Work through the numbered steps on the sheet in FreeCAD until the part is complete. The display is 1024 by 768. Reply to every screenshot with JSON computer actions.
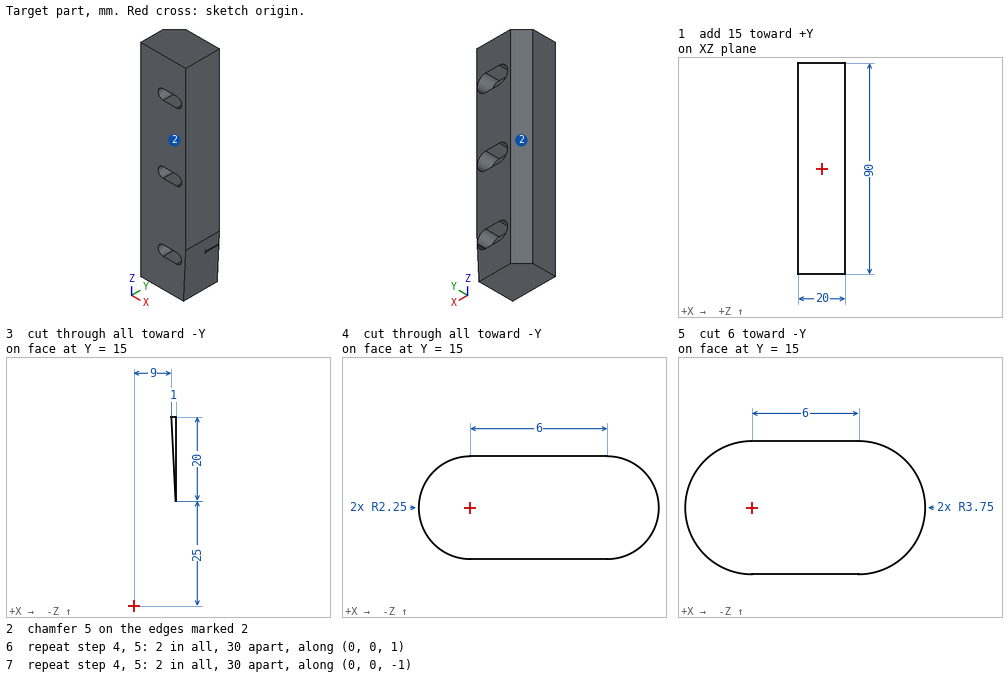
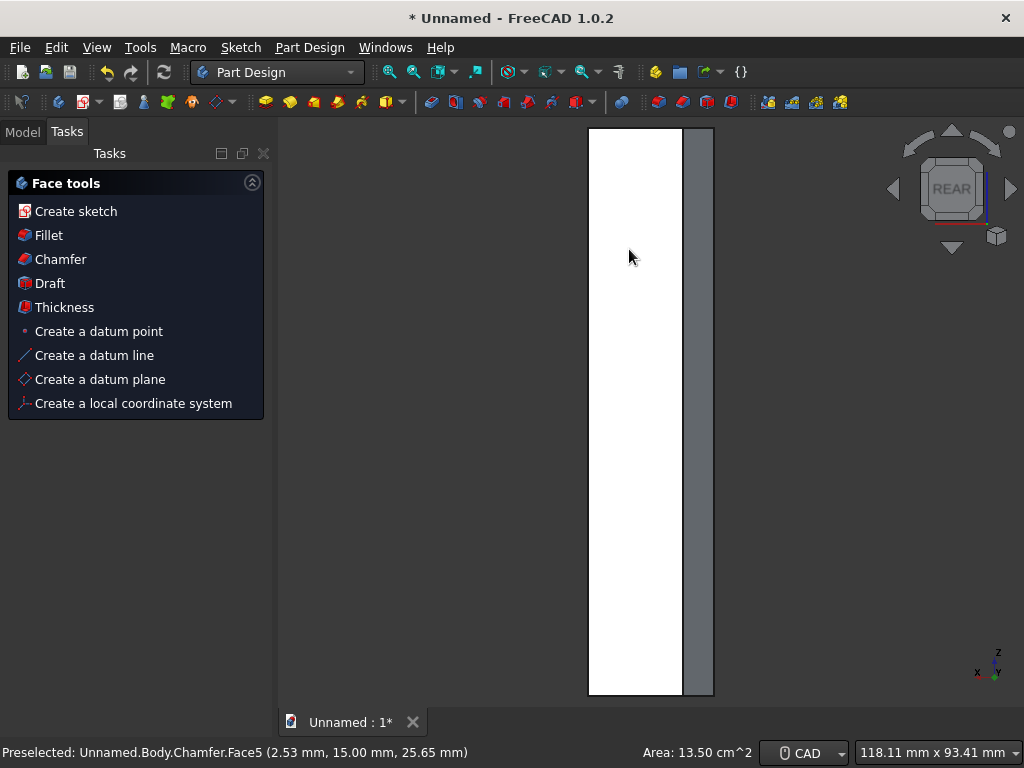
{"action": "left_click", "coordinate": [84, 102]}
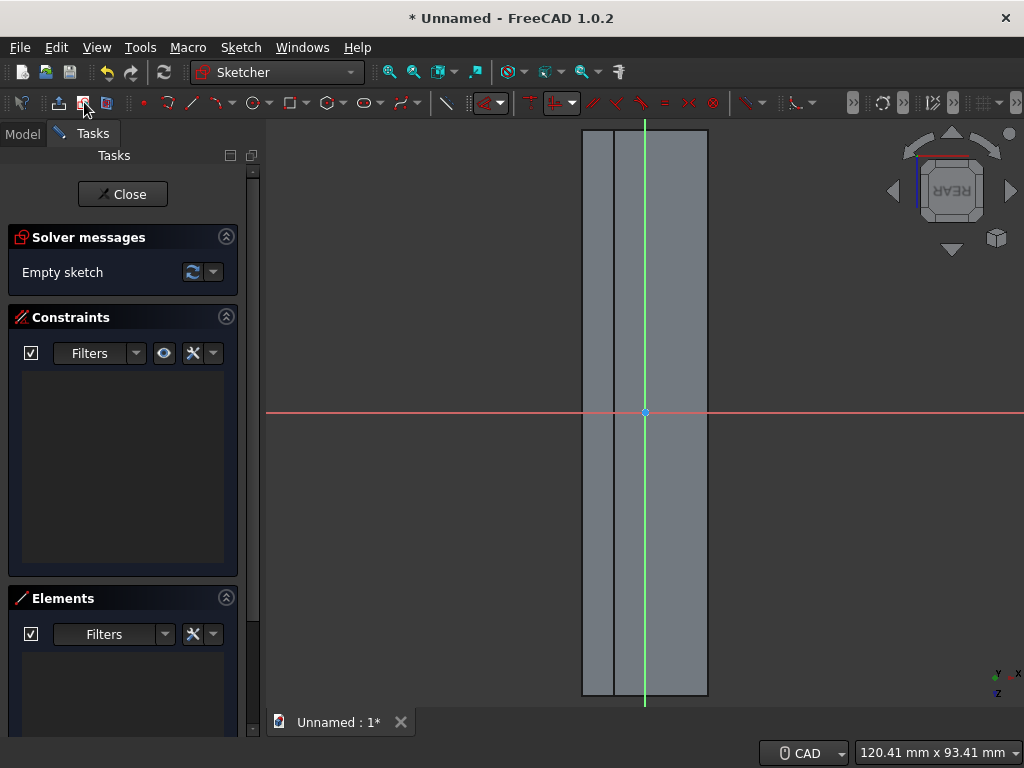
{"action": "scroll", "coordinate": [294, 679], "scroll_direction": "down", "scroll_amount": 1}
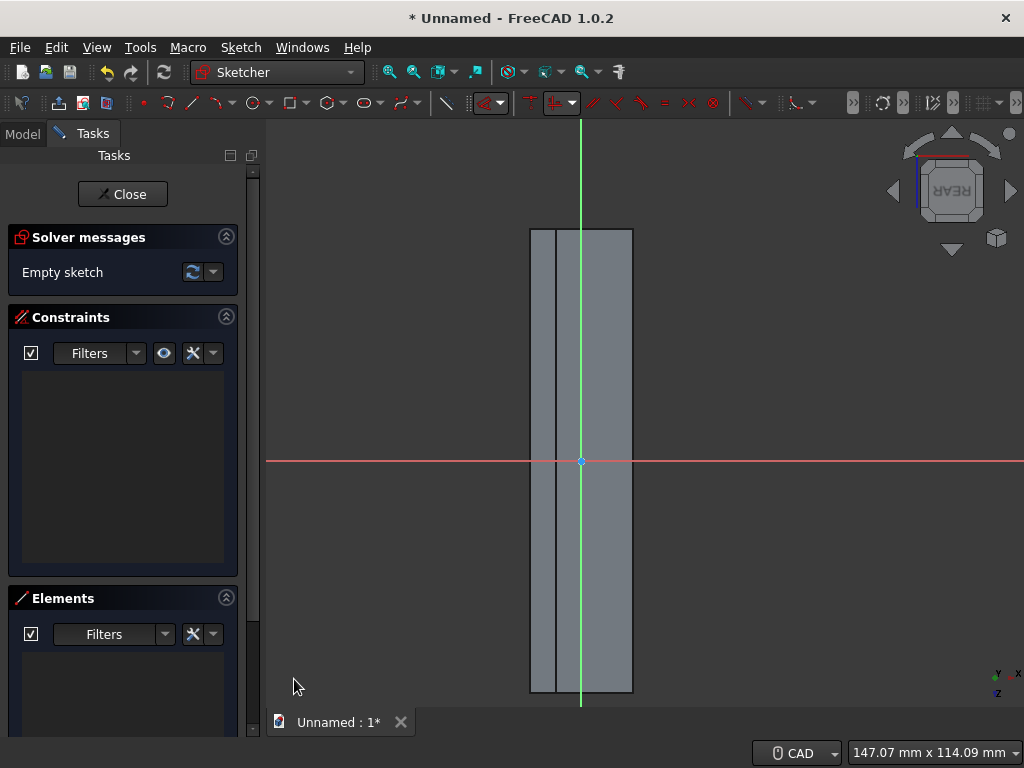
{"action": "scroll", "coordinate": [669, 208], "scroll_direction": "up", "scroll_amount": 2}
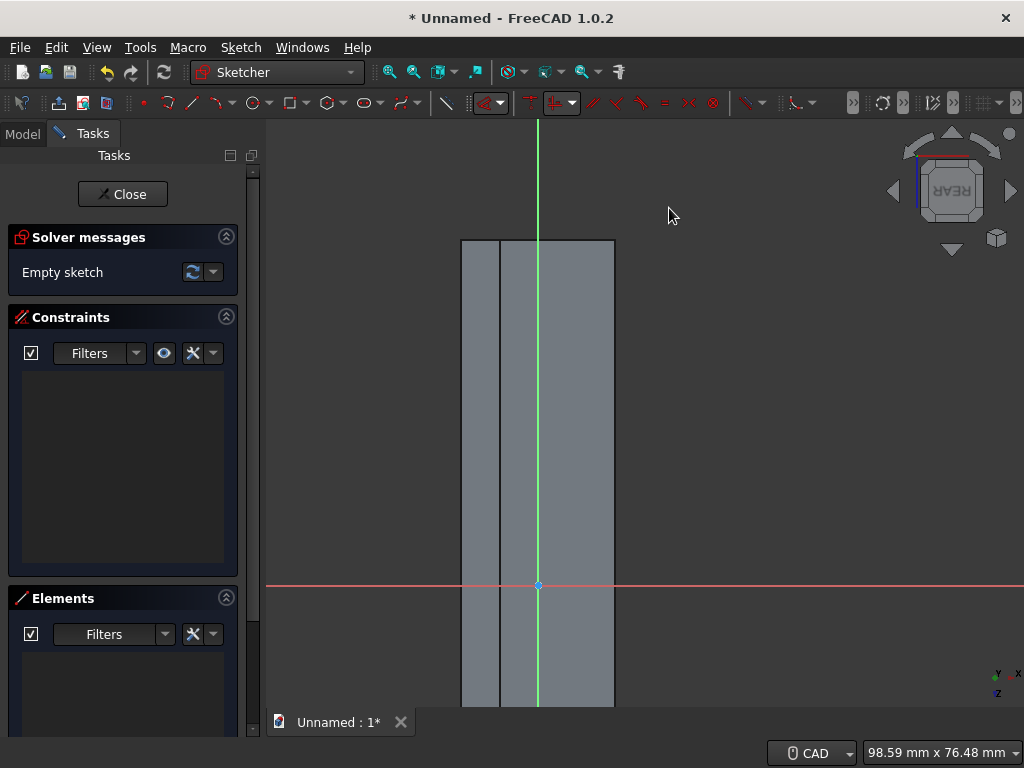
{"action": "left_click", "coordinate": [168, 104]}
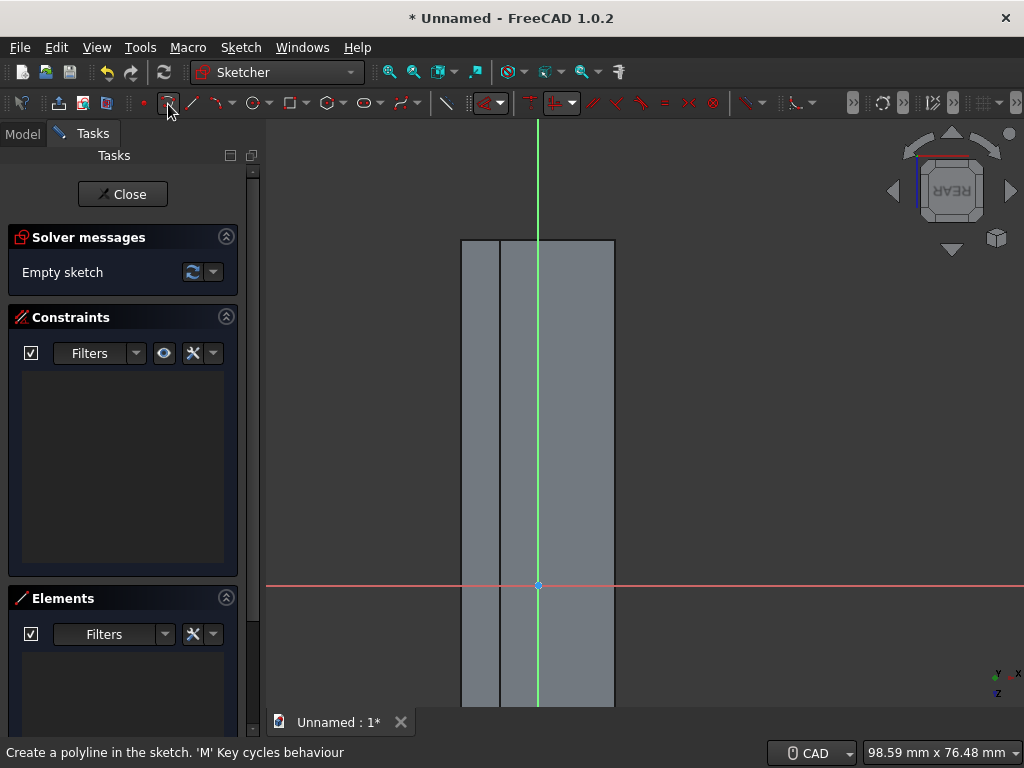
{"action": "left_click", "coordinate": [615, 394]}
{"action": "left_click", "coordinate": [615, 240]}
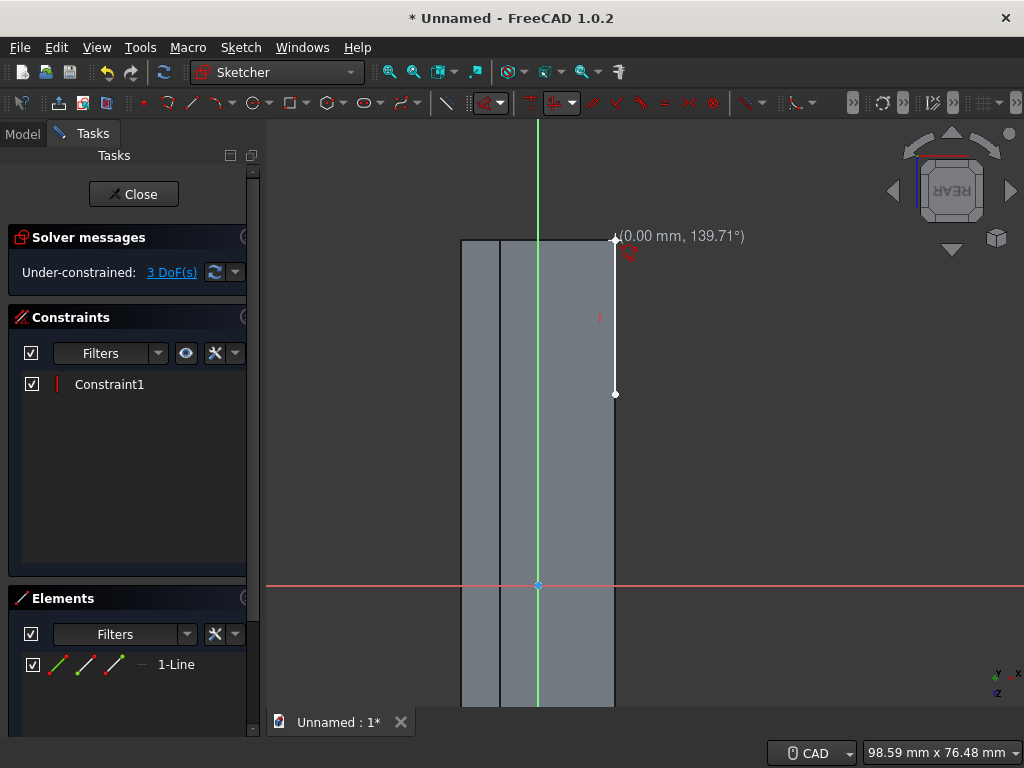
{"action": "scroll", "coordinate": [607, 240], "scroll_direction": "up", "scroll_amount": 4}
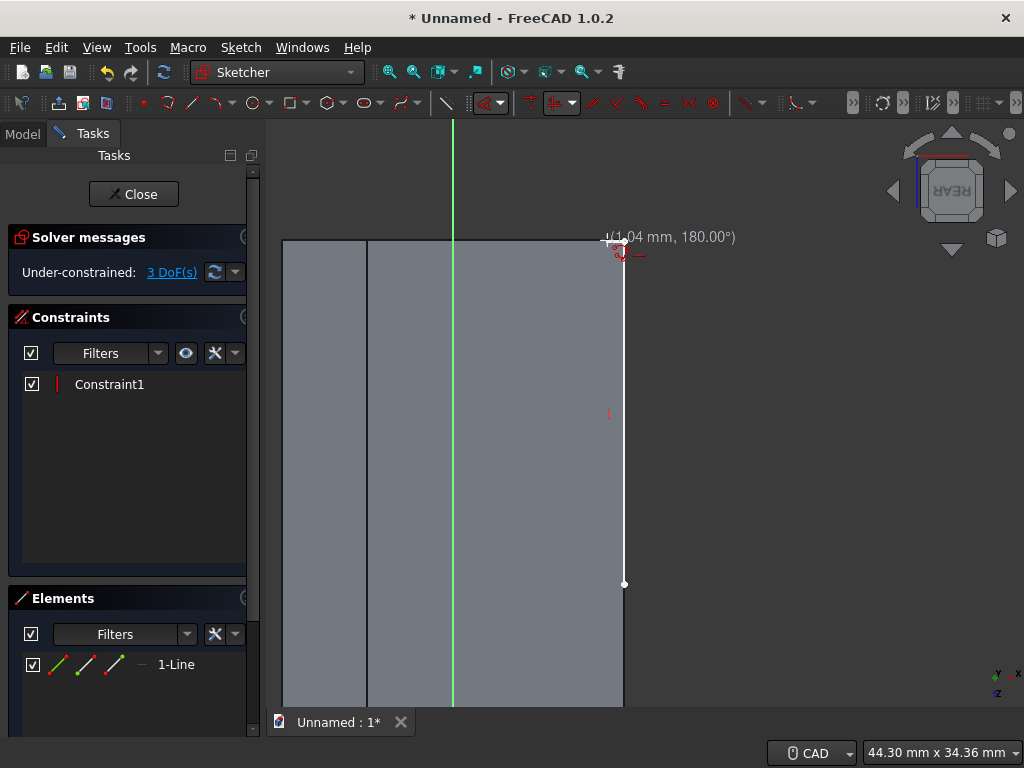
{"action": "left_click", "coordinate": [607, 240]}
{"action": "left_click", "coordinate": [624, 585]}
{"action": "key", "text": "Escape"}
{"action": "key", "text": "Escape"}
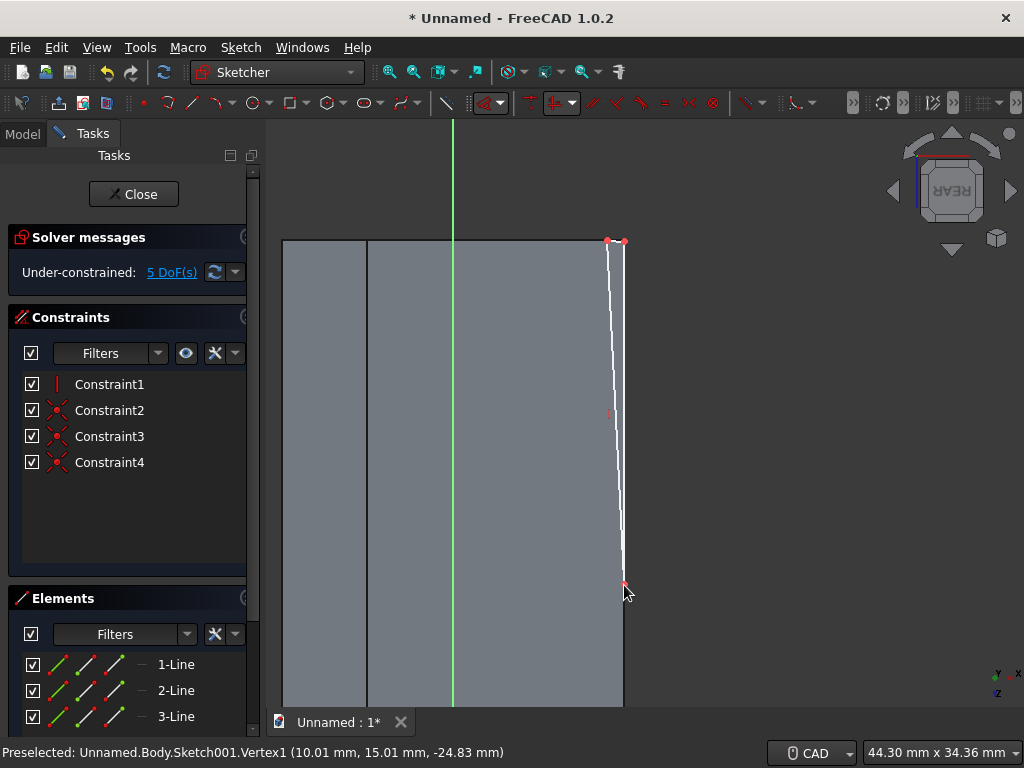
{"action": "scroll", "coordinate": [616, 241], "scroll_direction": "up", "scroll_amount": 3}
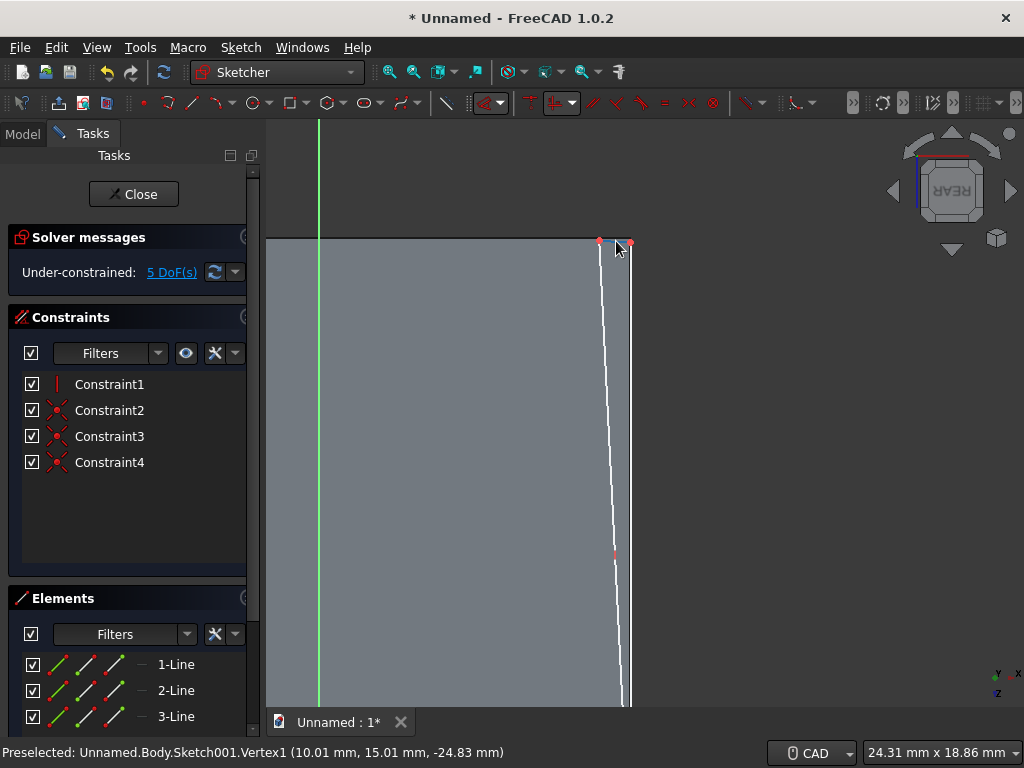
{"action": "left_click", "coordinate": [615, 242]}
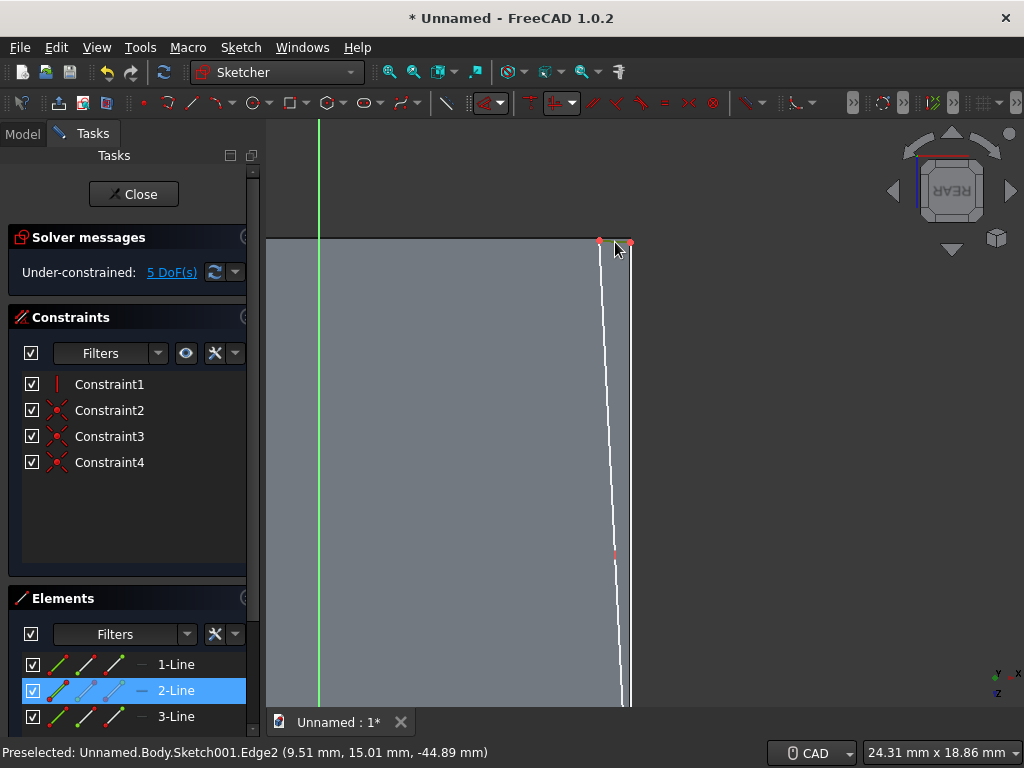
{"action": "left_click", "coordinate": [574, 104]}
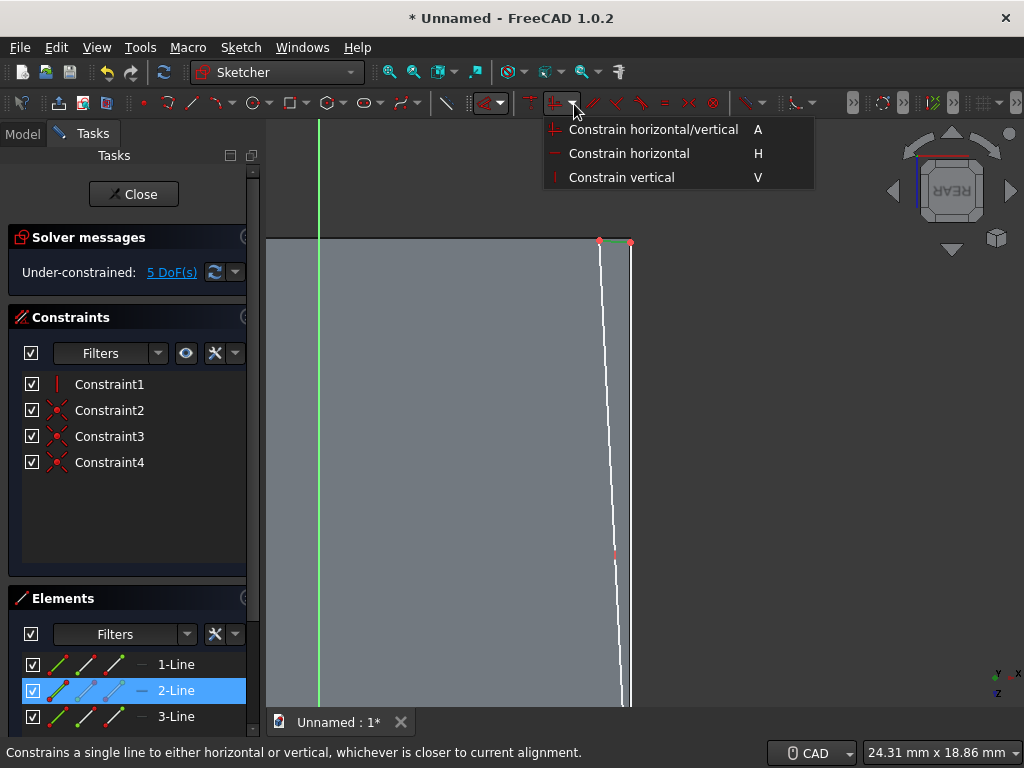
{"action": "left_click", "coordinate": [679, 153]}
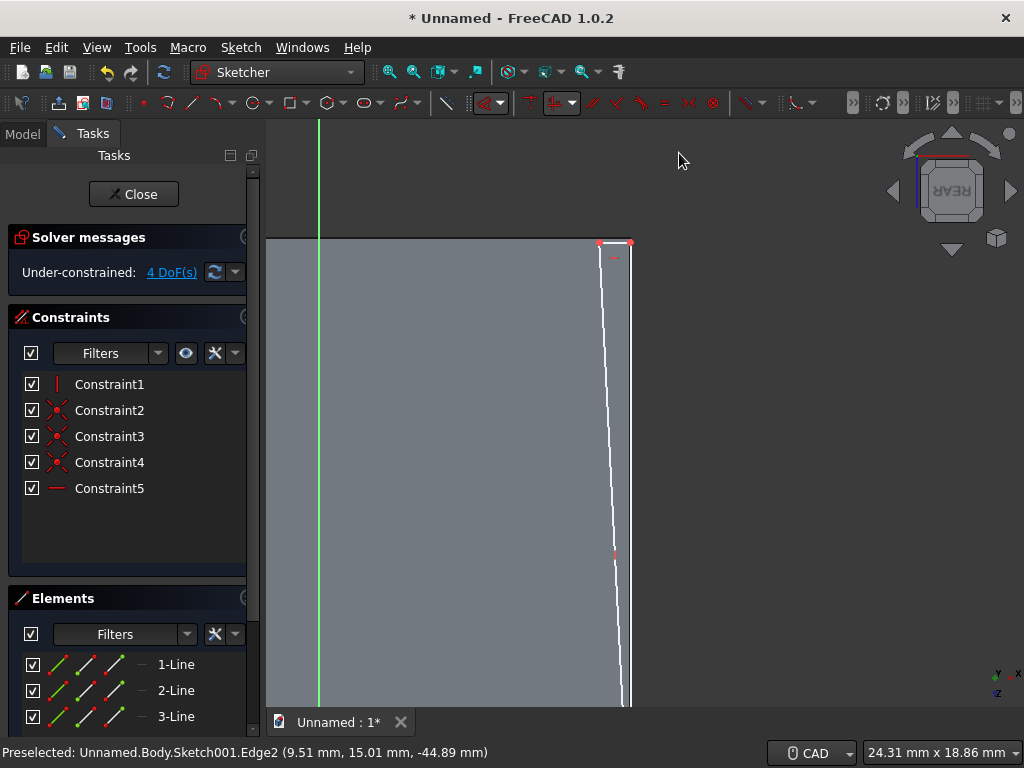
{"action": "scroll", "coordinate": [621, 243], "scroll_direction": "up", "scroll_amount": 2}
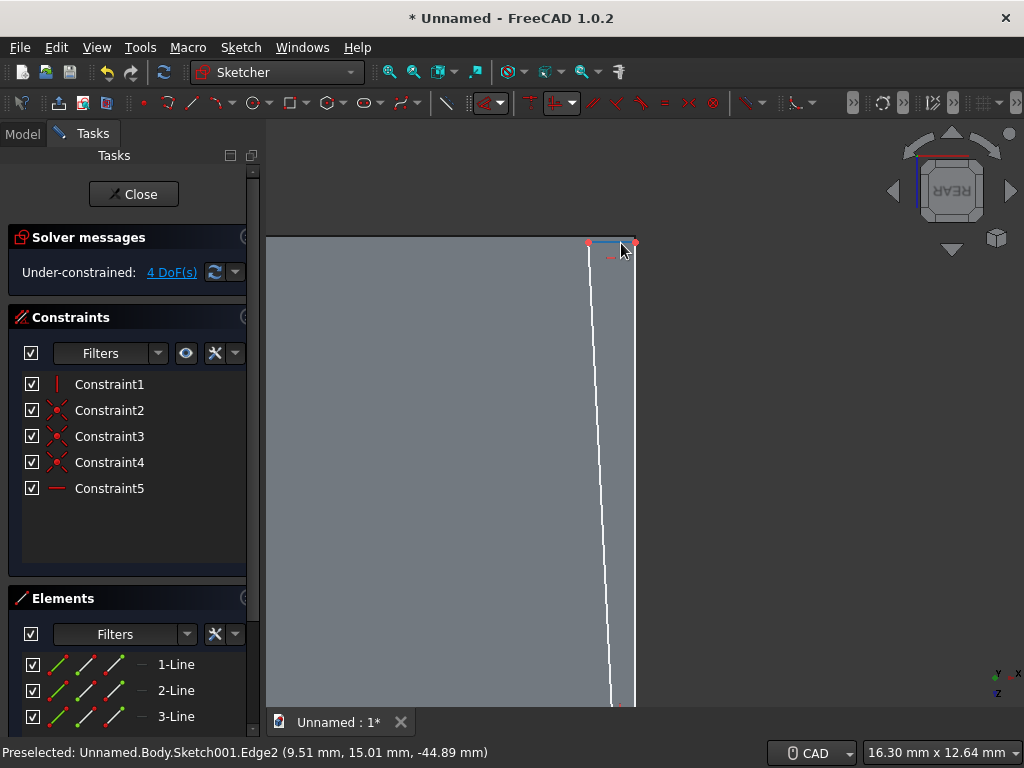
{"action": "left_click", "coordinate": [621, 242]}